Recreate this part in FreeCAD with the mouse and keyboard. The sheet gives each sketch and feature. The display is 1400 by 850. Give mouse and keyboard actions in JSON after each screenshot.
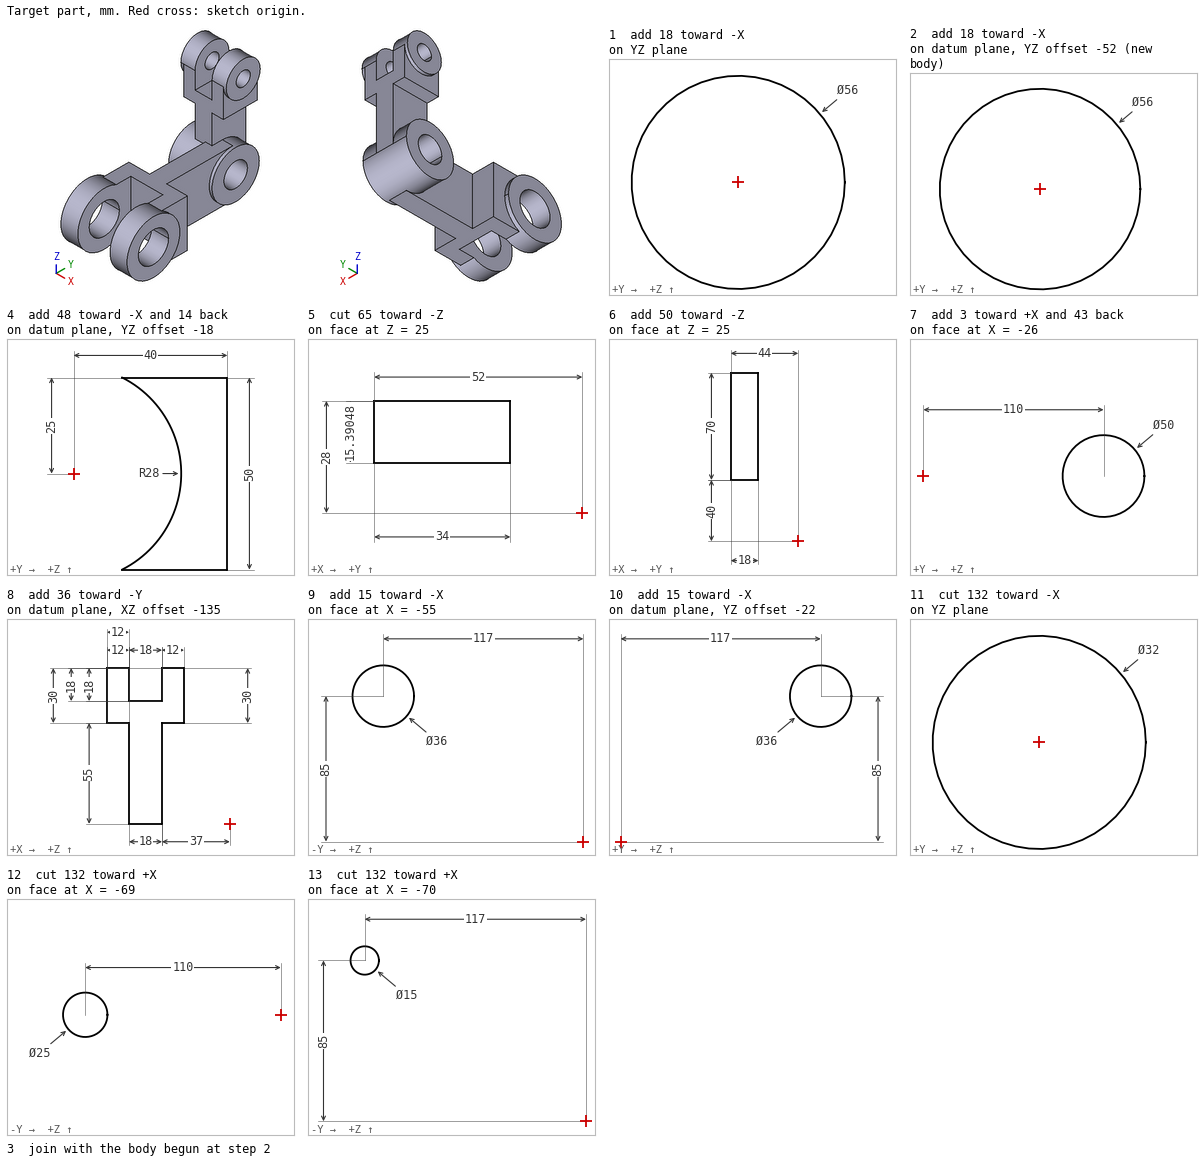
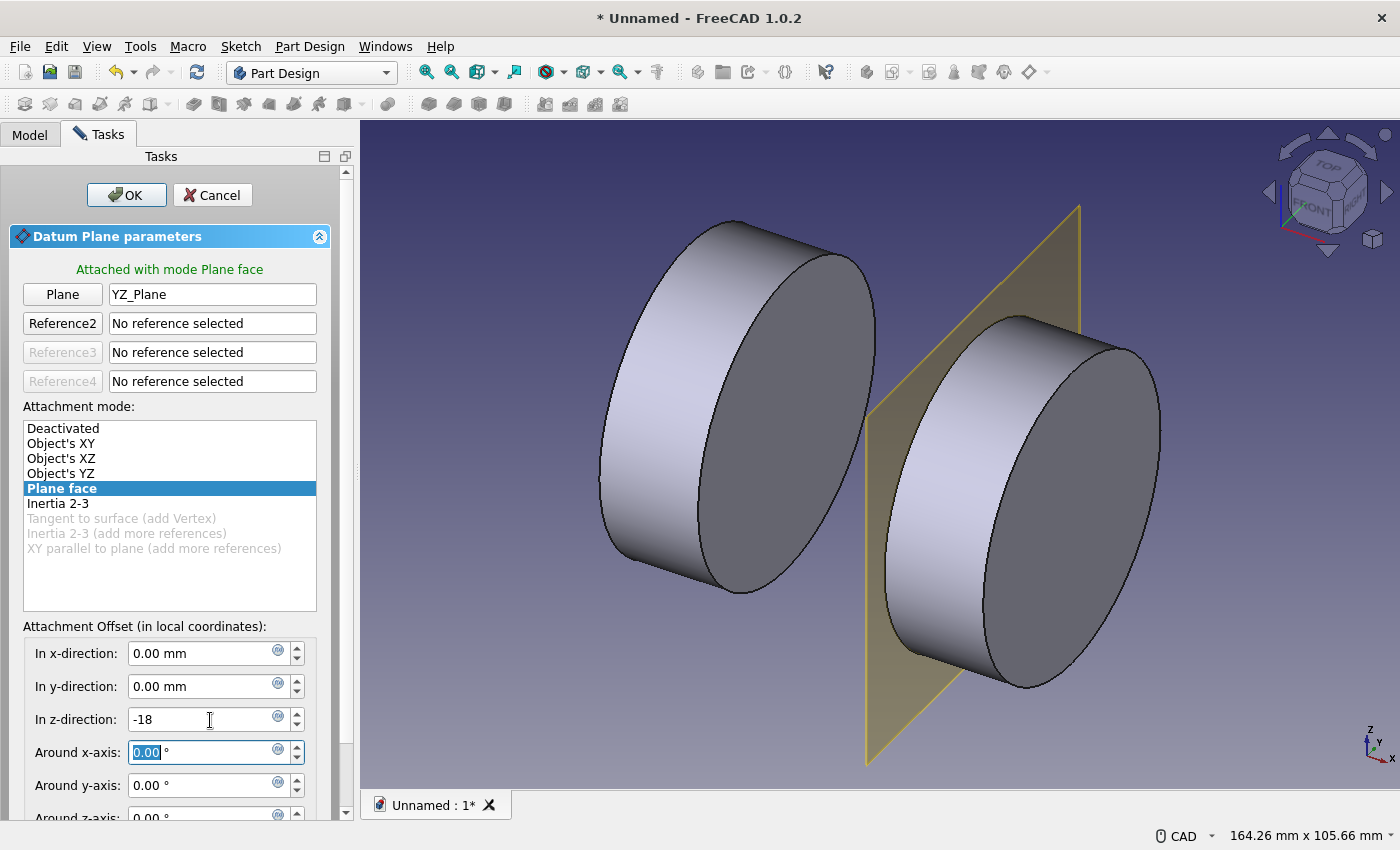
{"action": "left_click", "coordinate": [127, 195]}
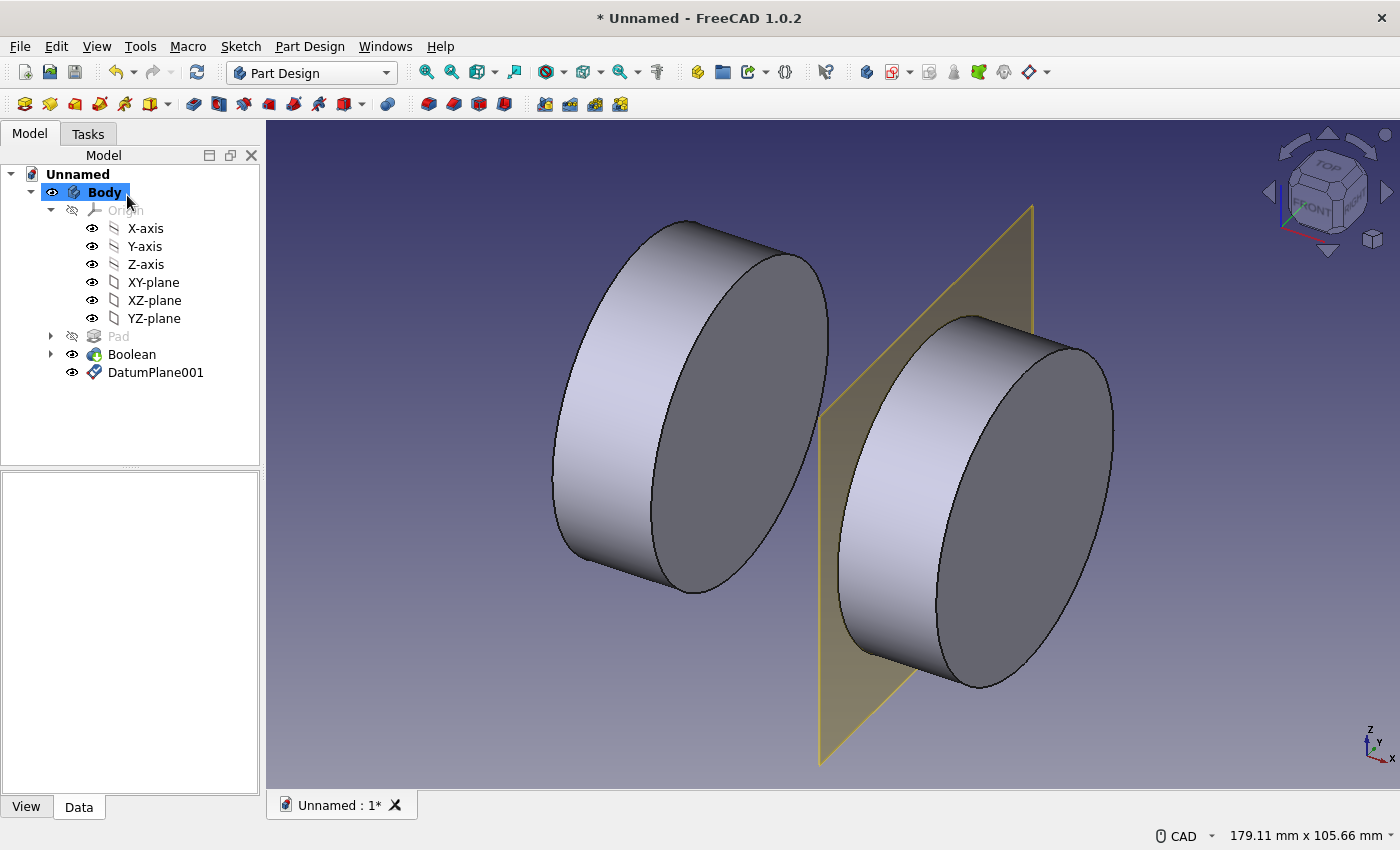
{"action": "left_click", "coordinate": [117, 372]}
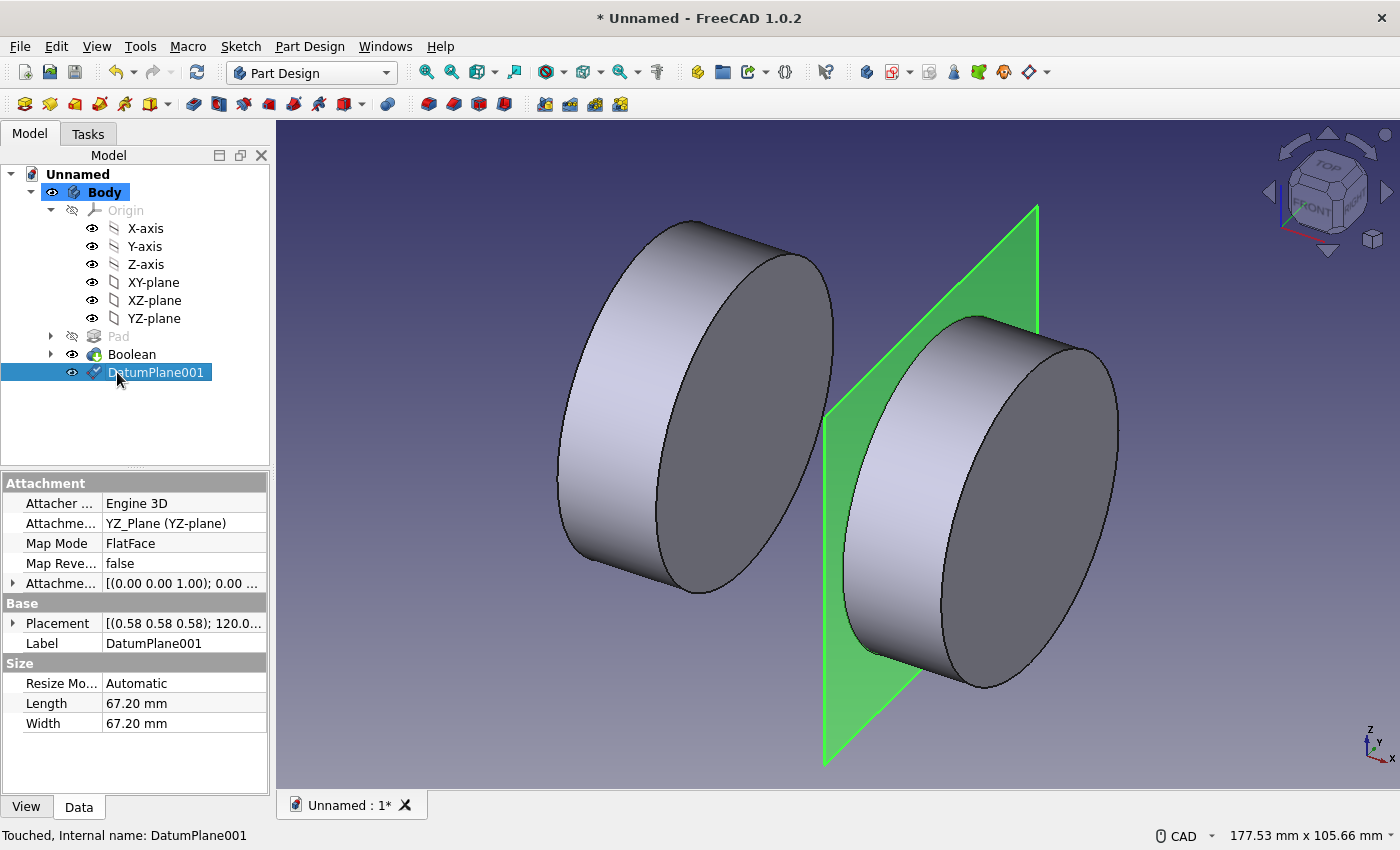
{"action": "left_click", "coordinate": [892, 72]}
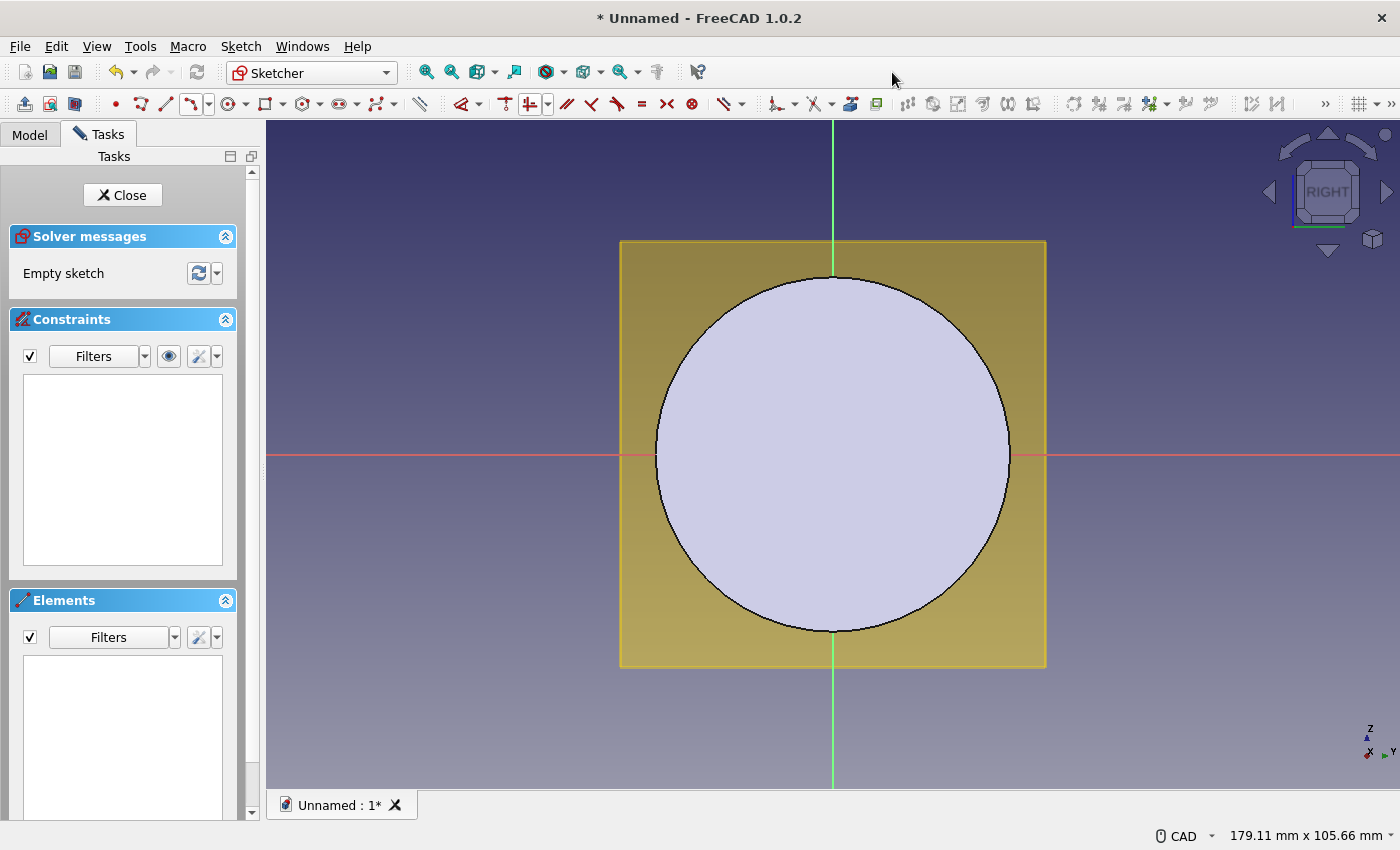
{"action": "key", "text": "q s"}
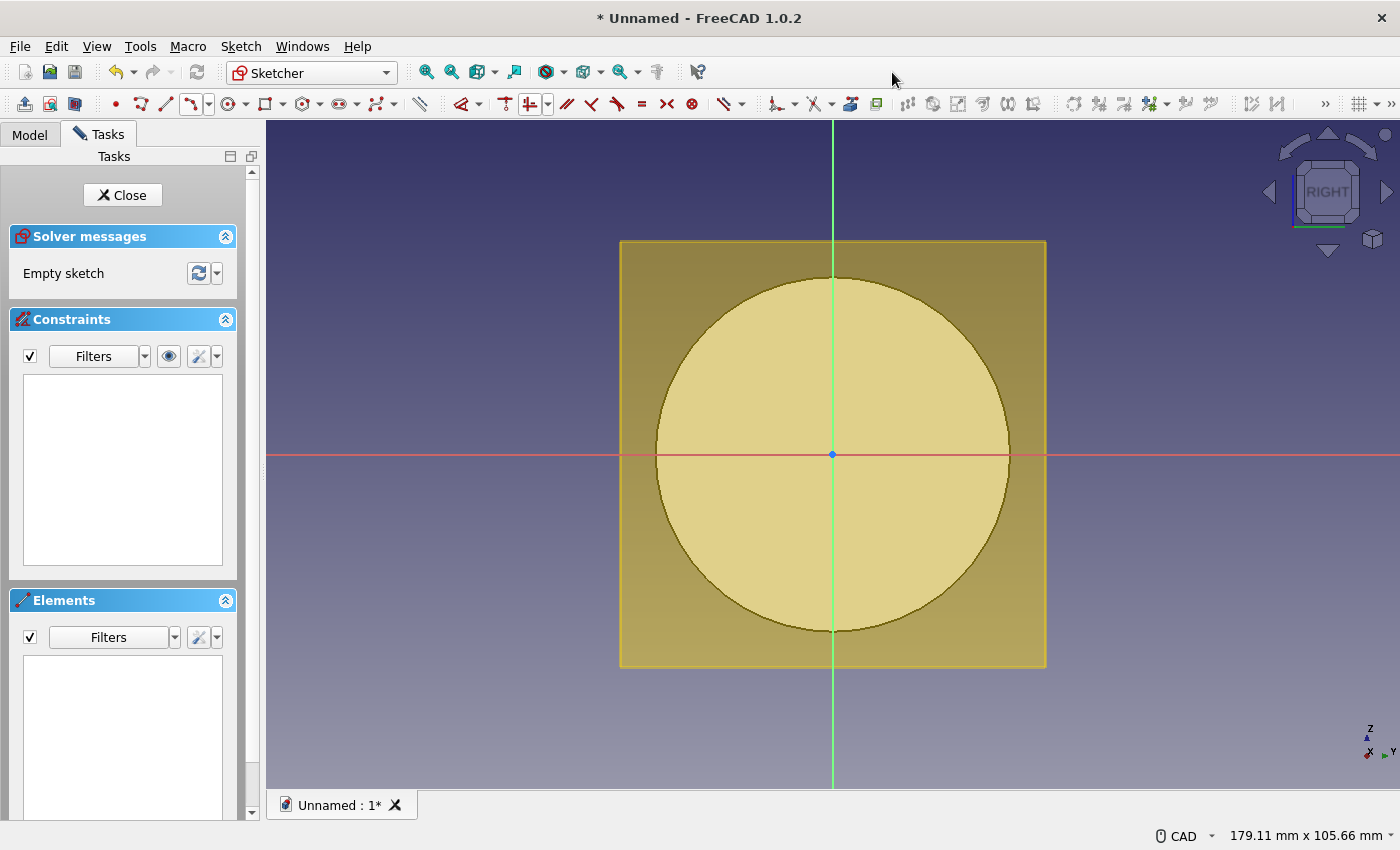
{"action": "scroll", "coordinate": [1235, 455], "scroll_direction": "up", "scroll_amount": 2}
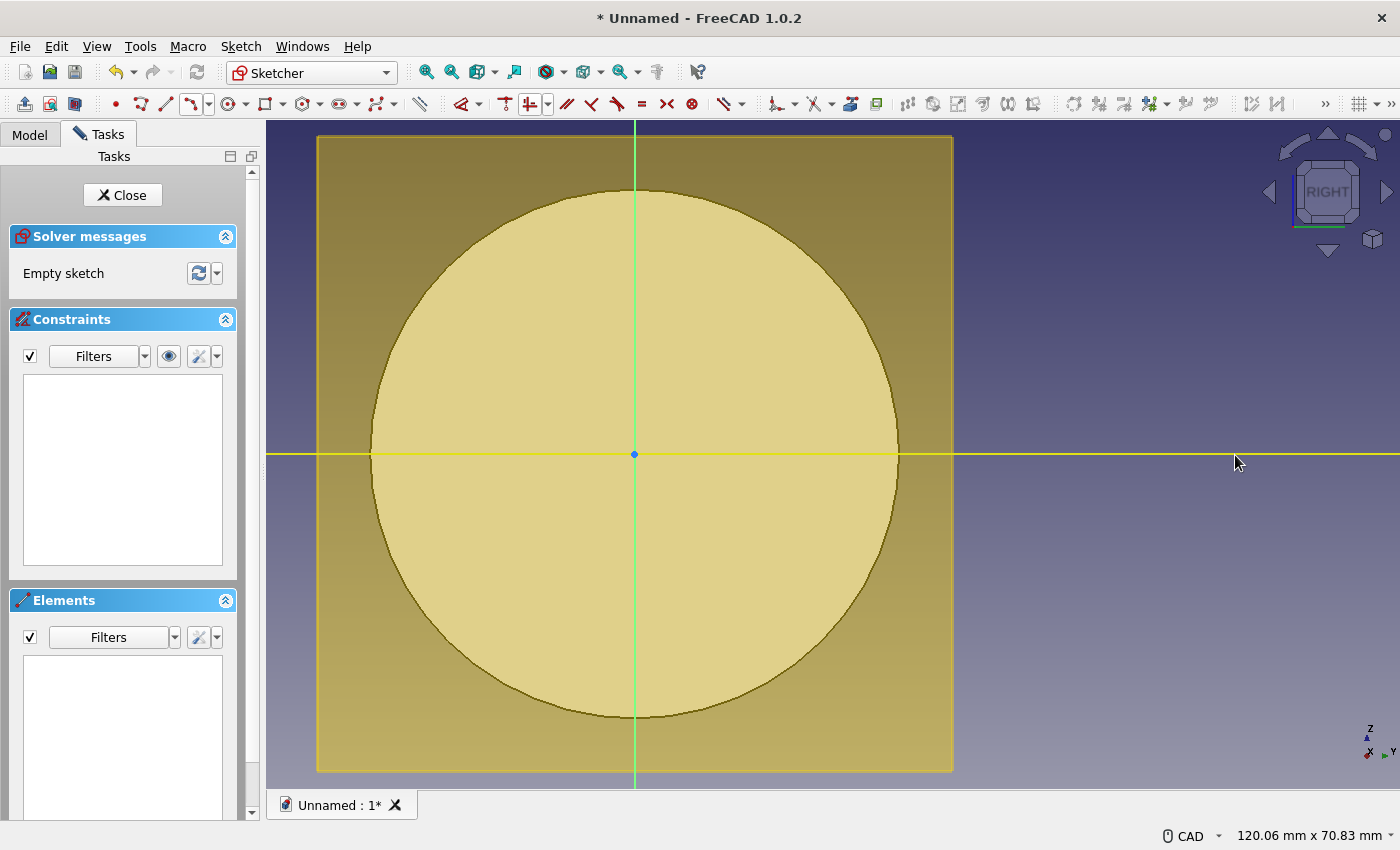
{"action": "left_click", "coordinate": [141, 104]}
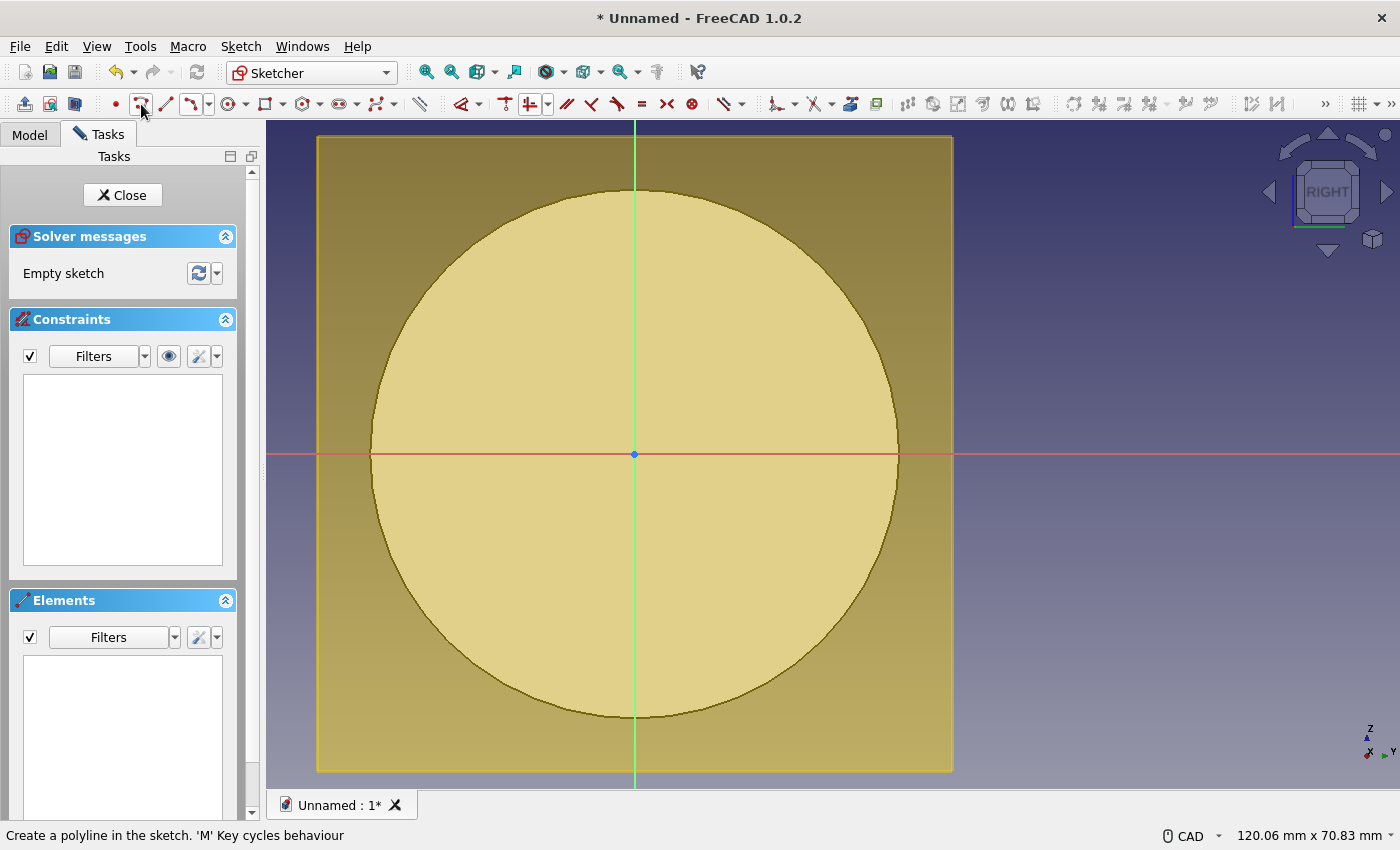
{"action": "left_click", "coordinate": [754, 218]}
{"action": "left_click", "coordinate": [1012, 218]}
{"action": "left_click", "coordinate": [1012, 690]}
{"action": "left_click", "coordinate": [754, 690]}
{"action": "right_click", "coordinate": [754, 690]}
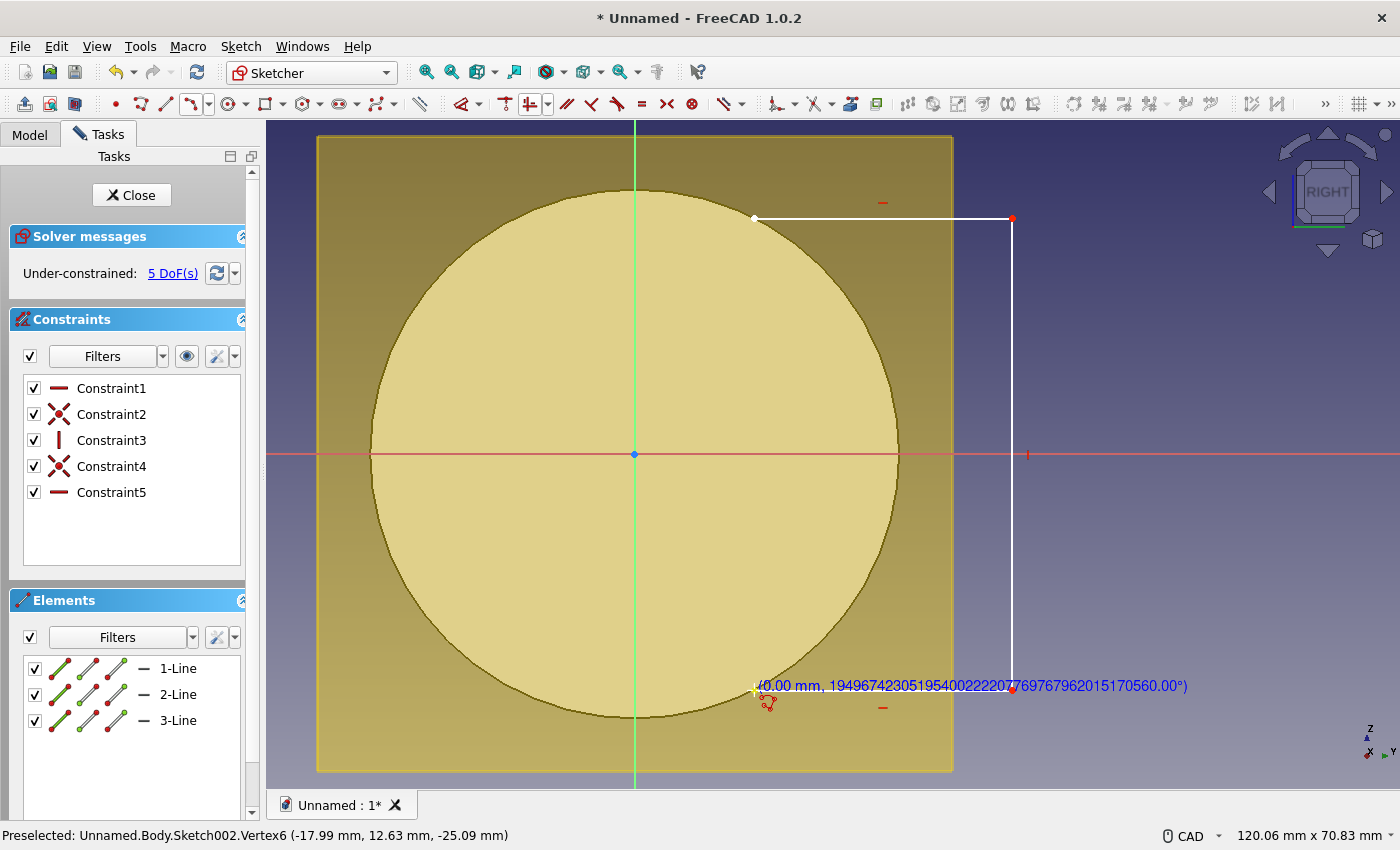
{"action": "left_click", "coordinate": [190, 104]}